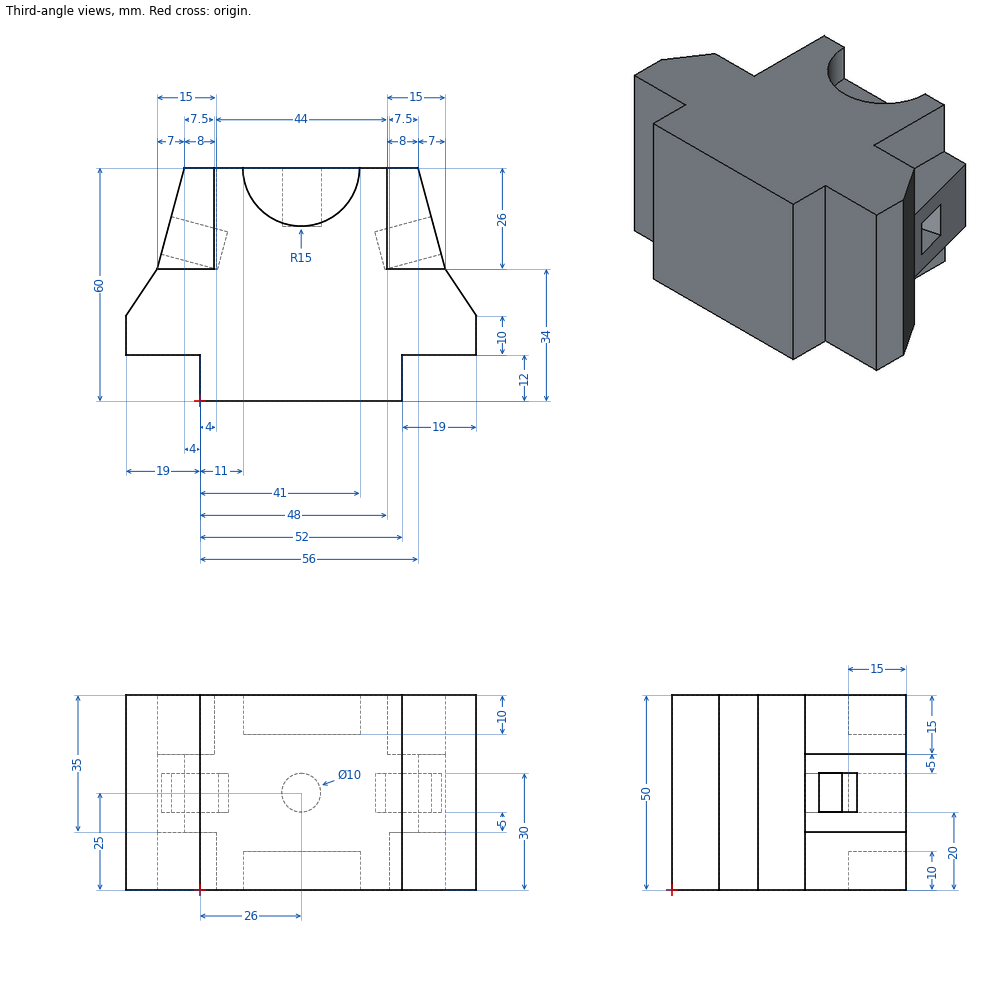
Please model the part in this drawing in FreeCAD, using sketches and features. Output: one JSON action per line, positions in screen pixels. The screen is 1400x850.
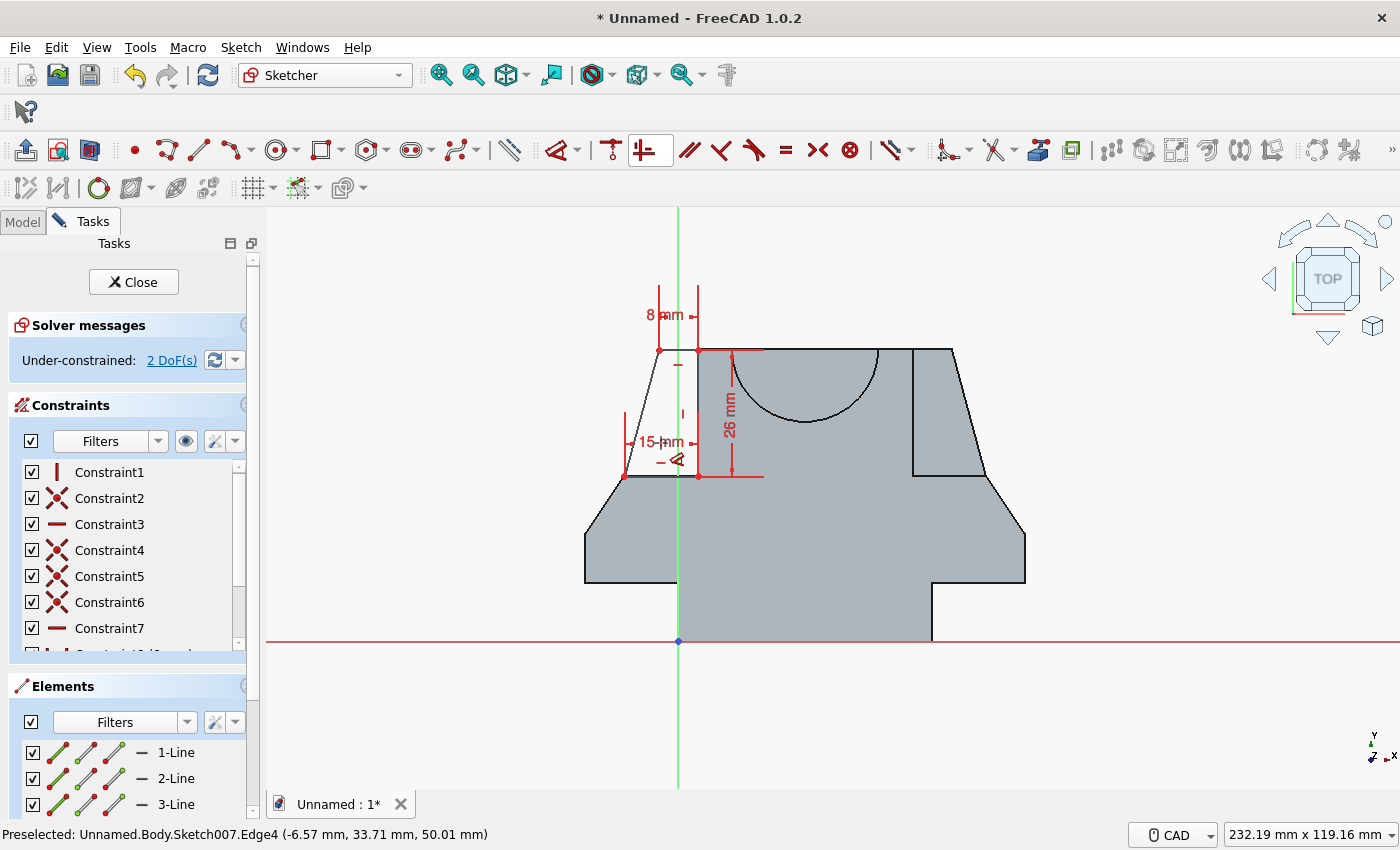
{"action": "scroll", "coordinate": [698, 477], "scroll_direction": "up", "scroll_amount": 4}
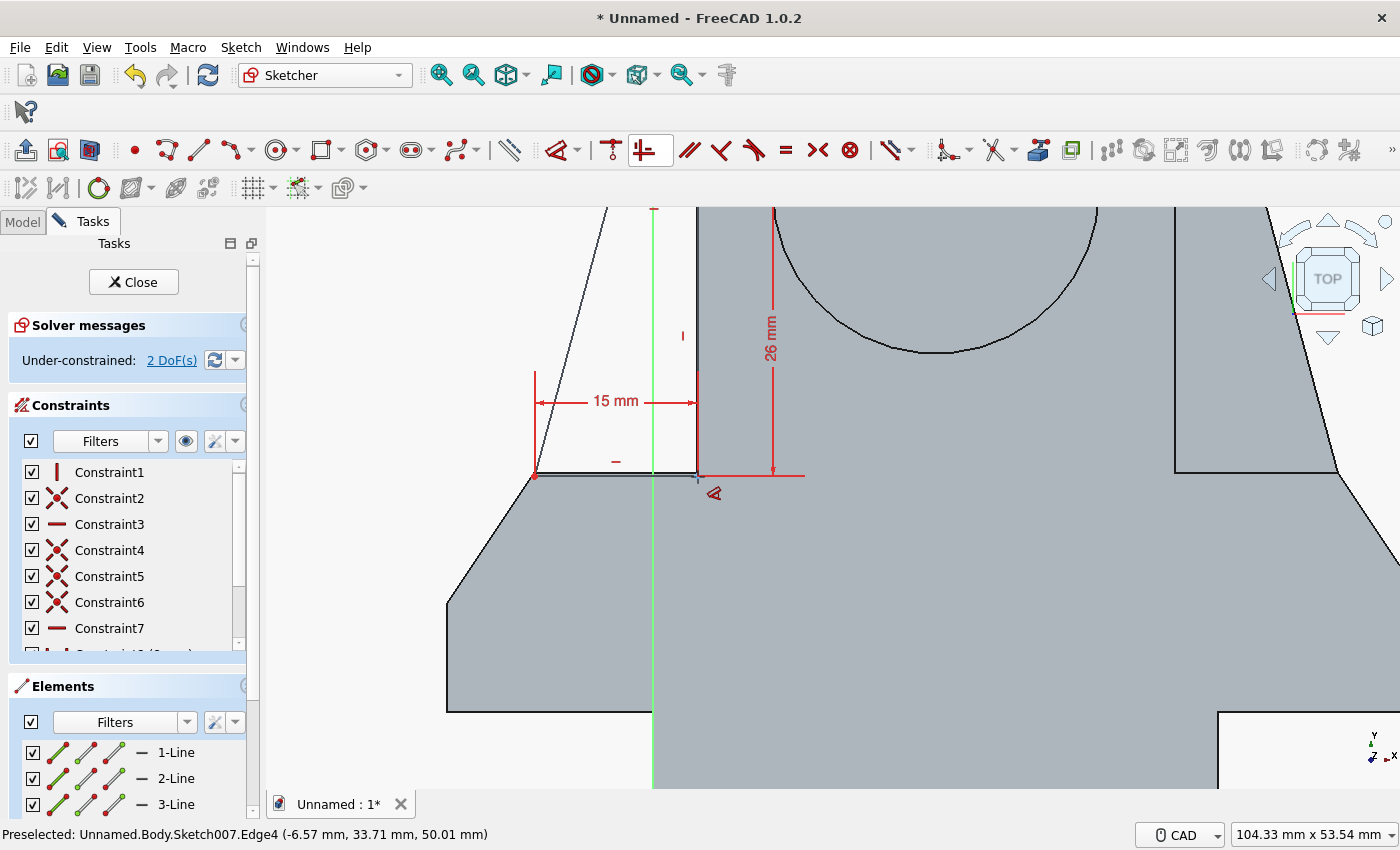
{"action": "left_click", "coordinate": [698, 476]}
{"action": "left_click", "coordinate": [675, 442]}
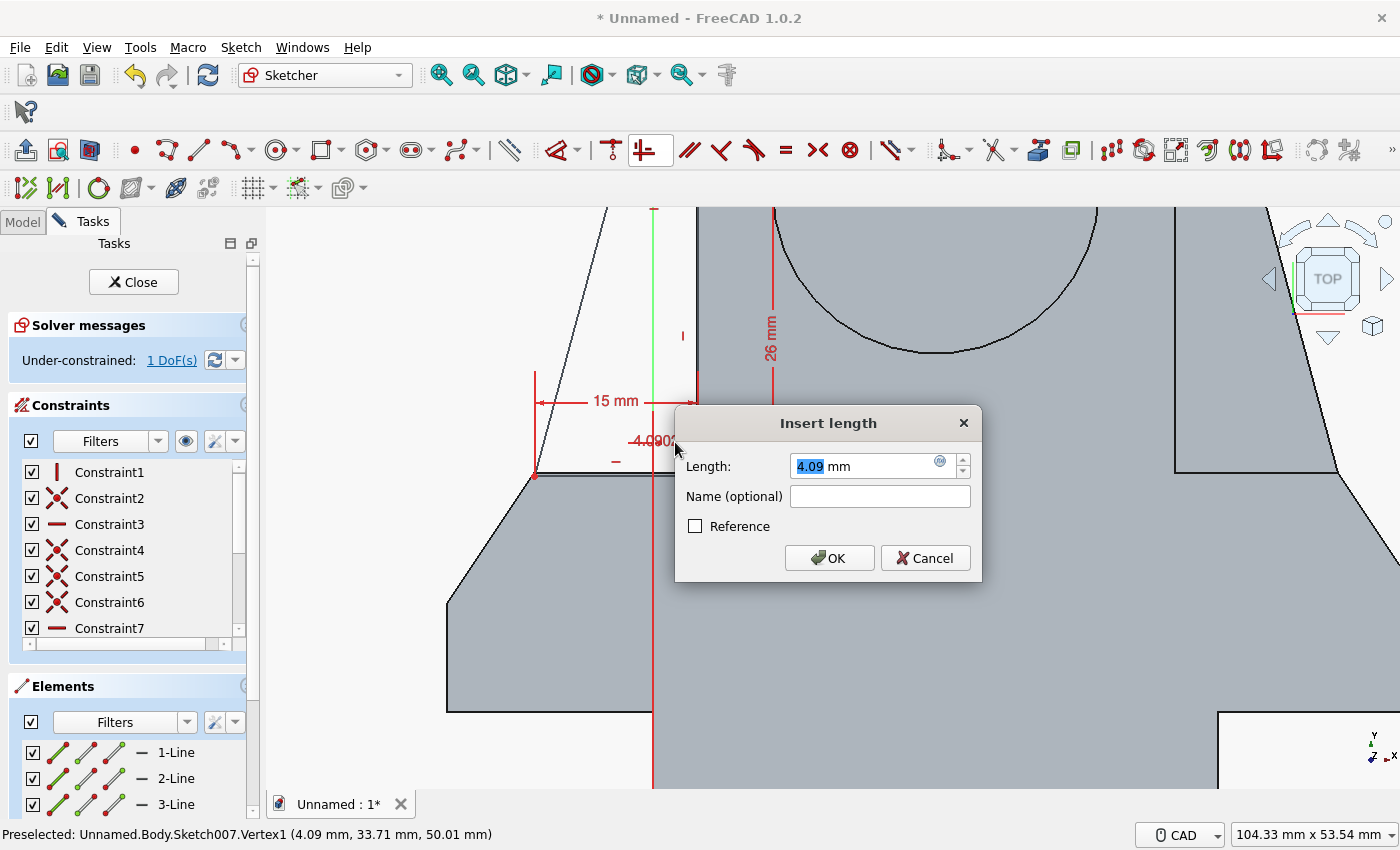
{"action": "type", "text": "4"}
{"action": "key", "text": "Return"}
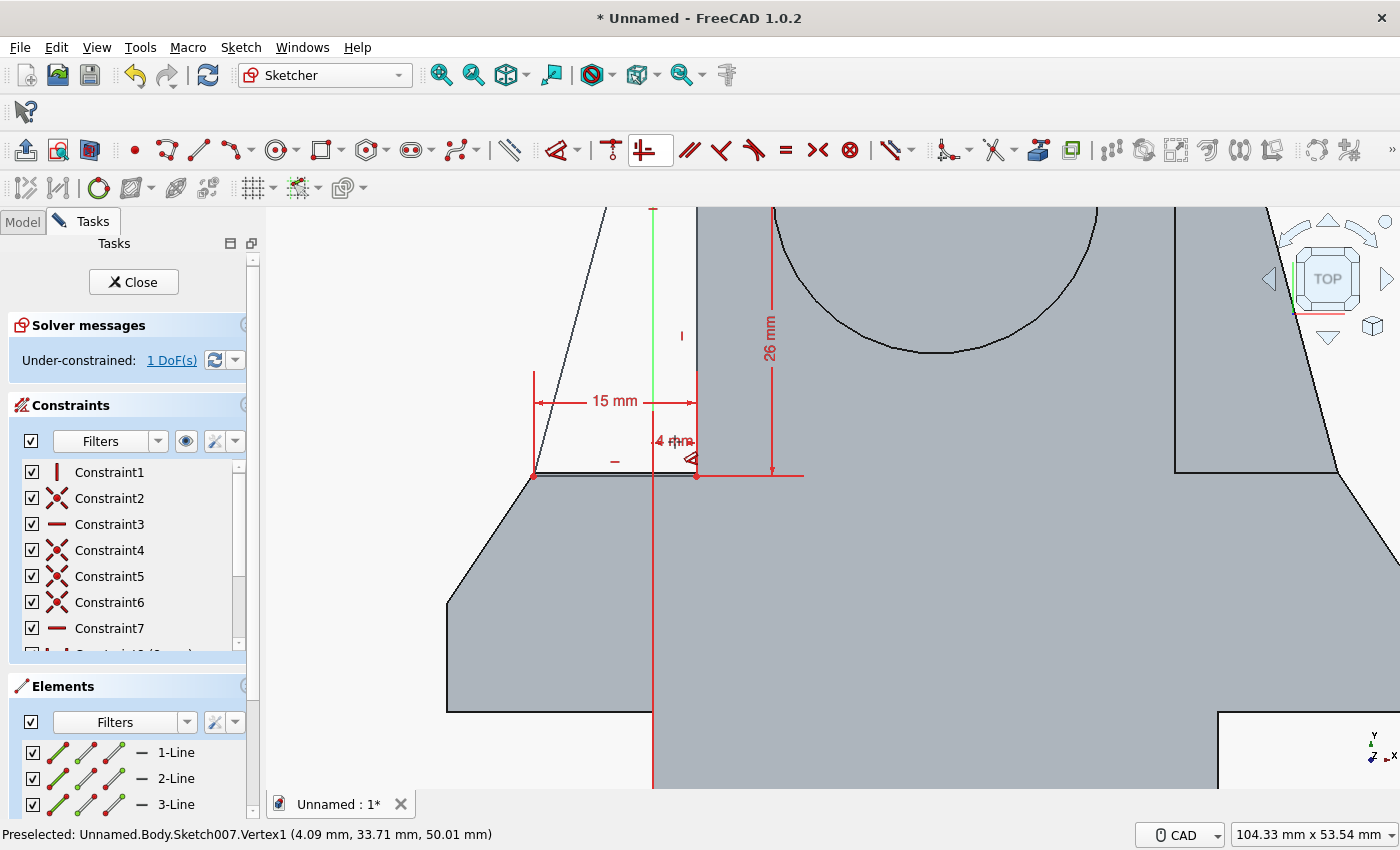
{"action": "left_click", "coordinate": [697, 476]}
{"action": "left_click", "coordinate": [731, 619]}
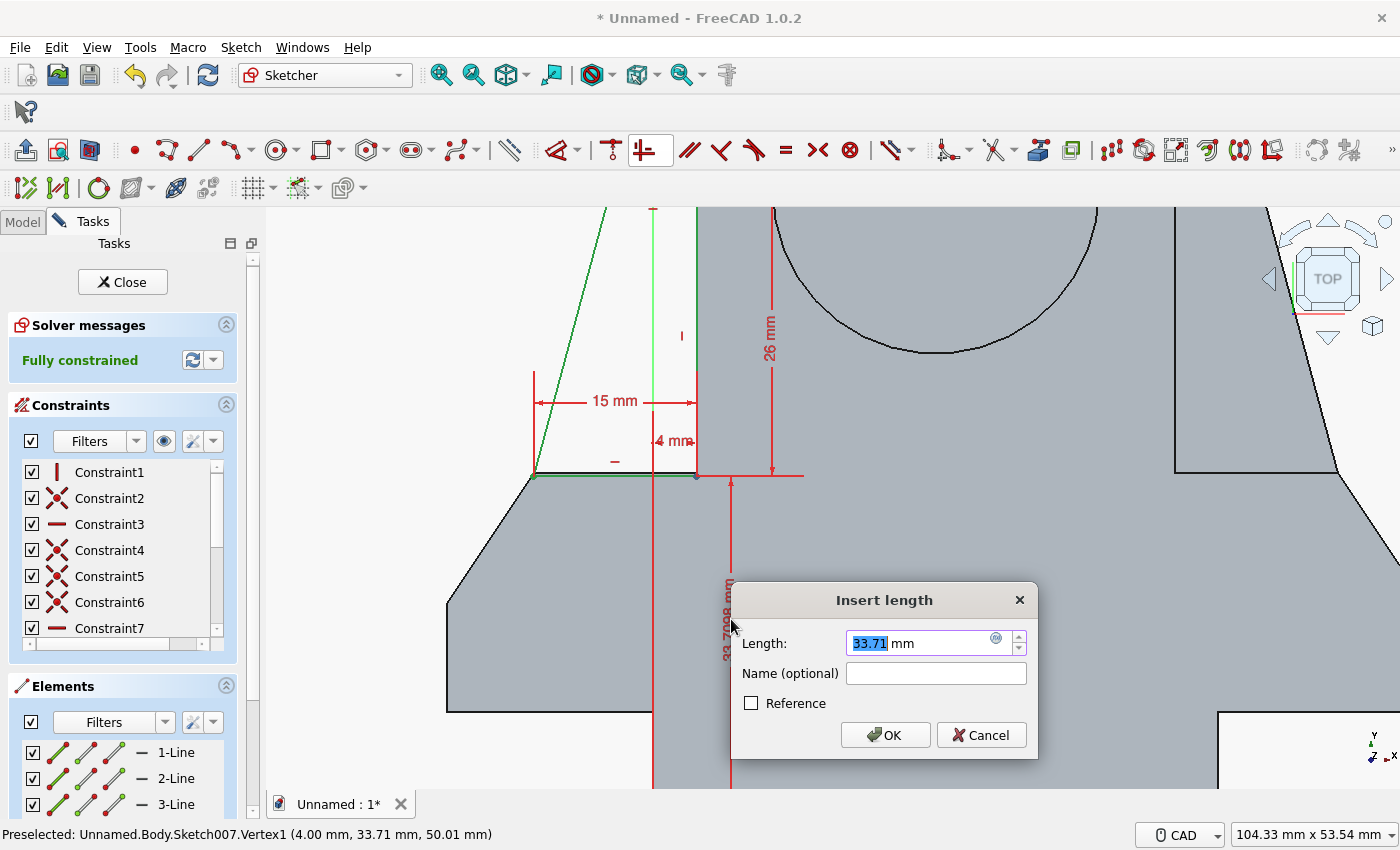
{"action": "type", "text": "34"}
{"action": "key", "text": "Return"}
{"action": "key", "text": "Escape"}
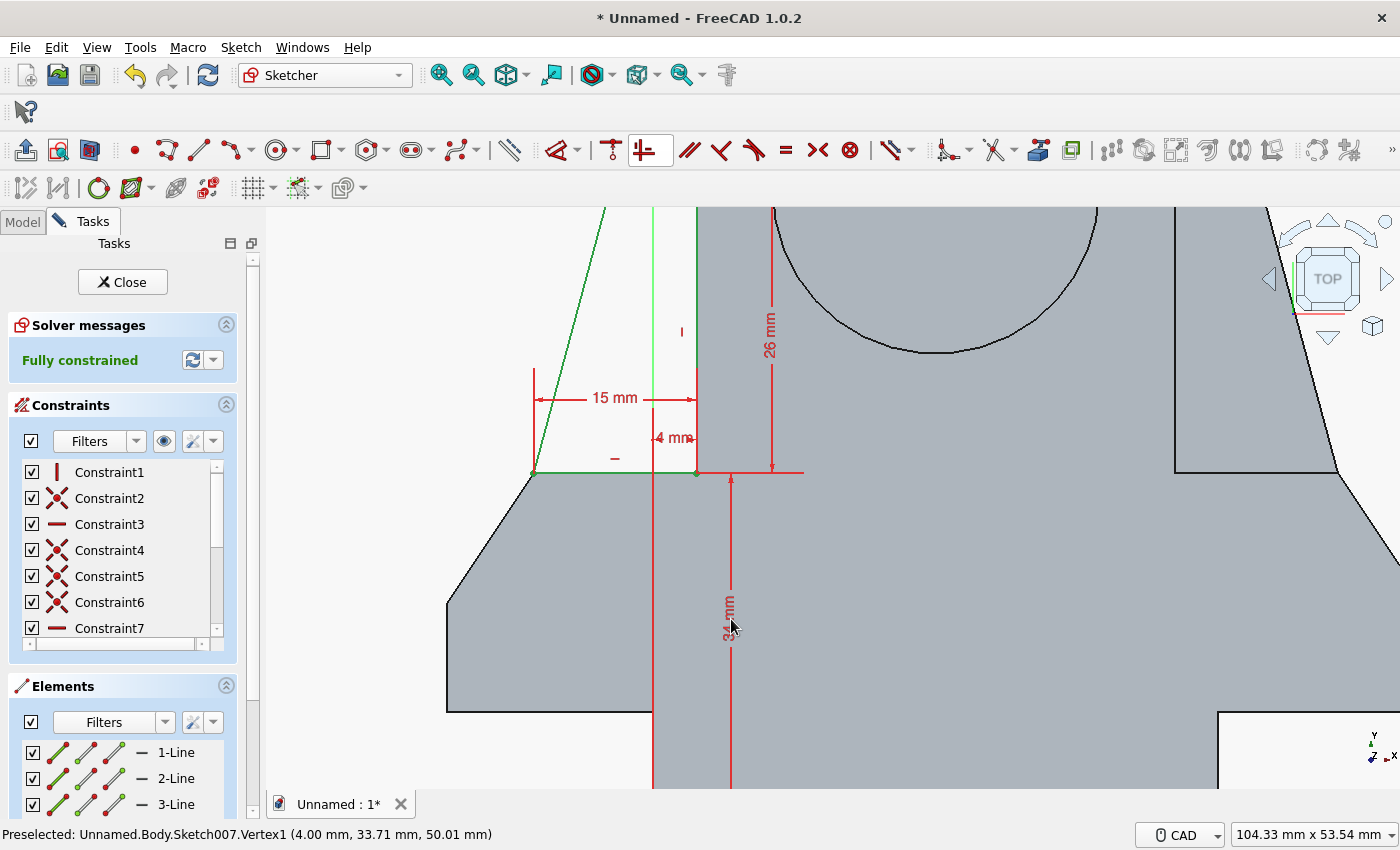
{"action": "left_click", "coordinate": [123, 282]}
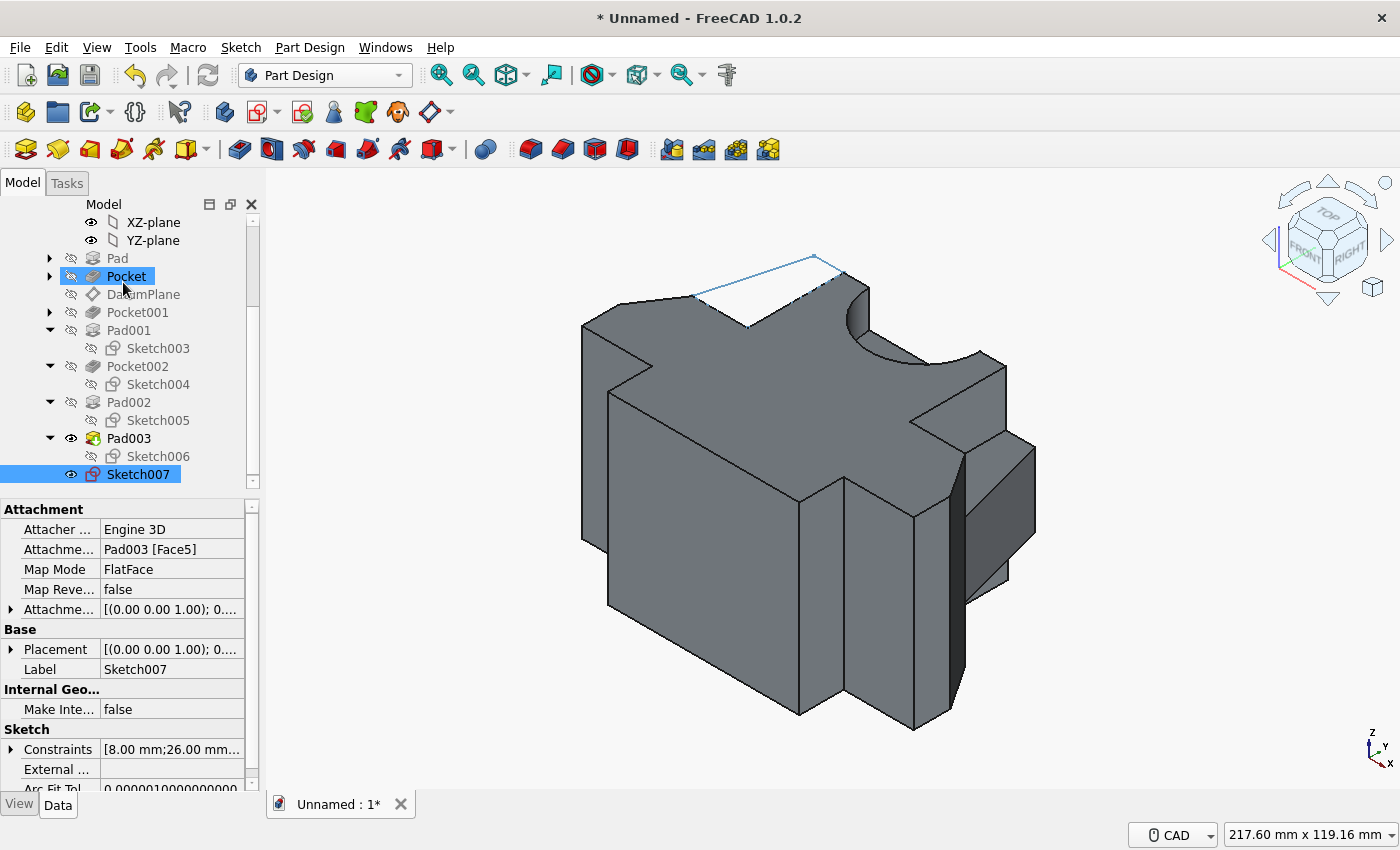
{"action": "left_click", "coordinate": [26, 150]}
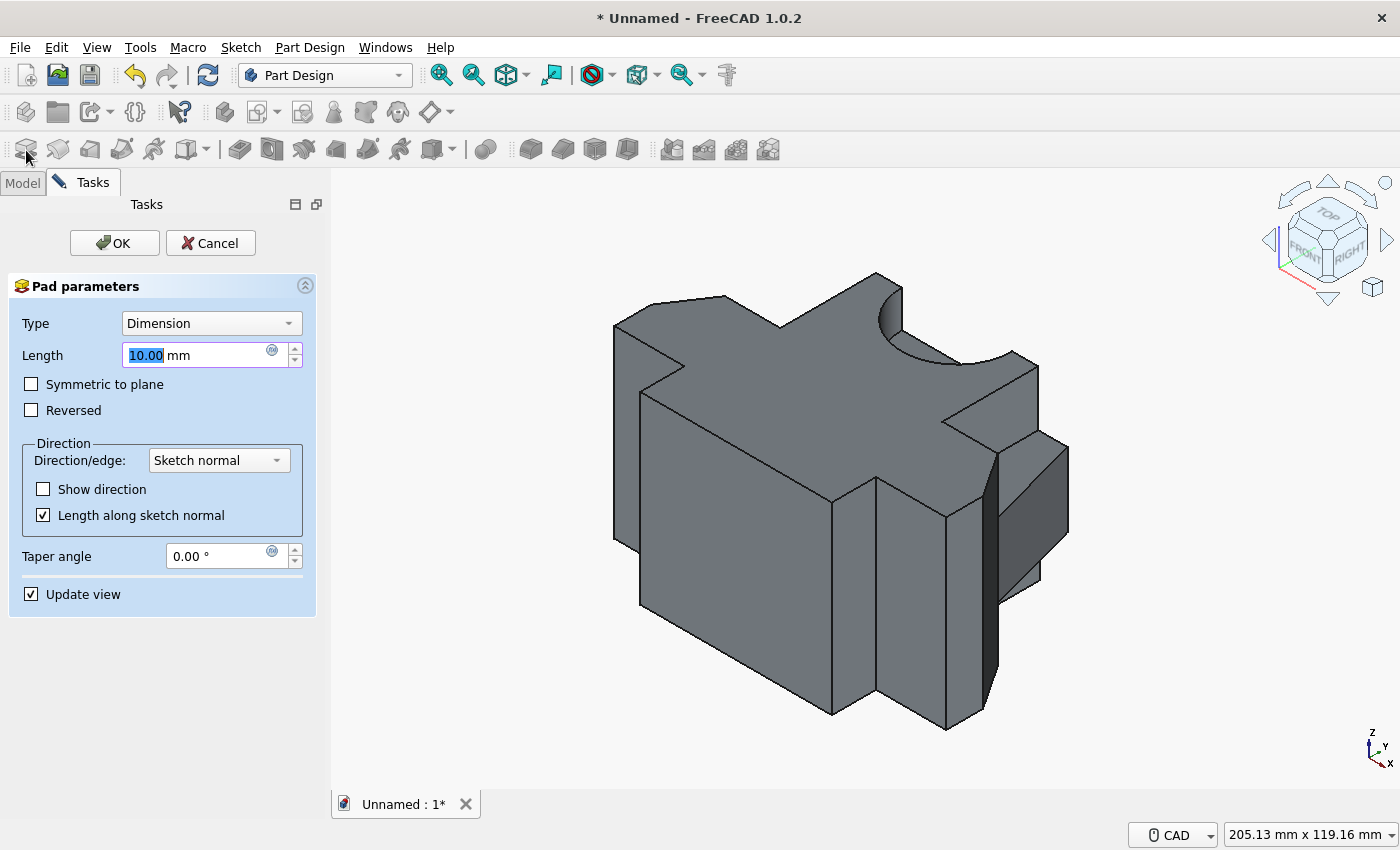
{"action": "type", "text": "35"}
{"action": "key", "text": "Tab"}